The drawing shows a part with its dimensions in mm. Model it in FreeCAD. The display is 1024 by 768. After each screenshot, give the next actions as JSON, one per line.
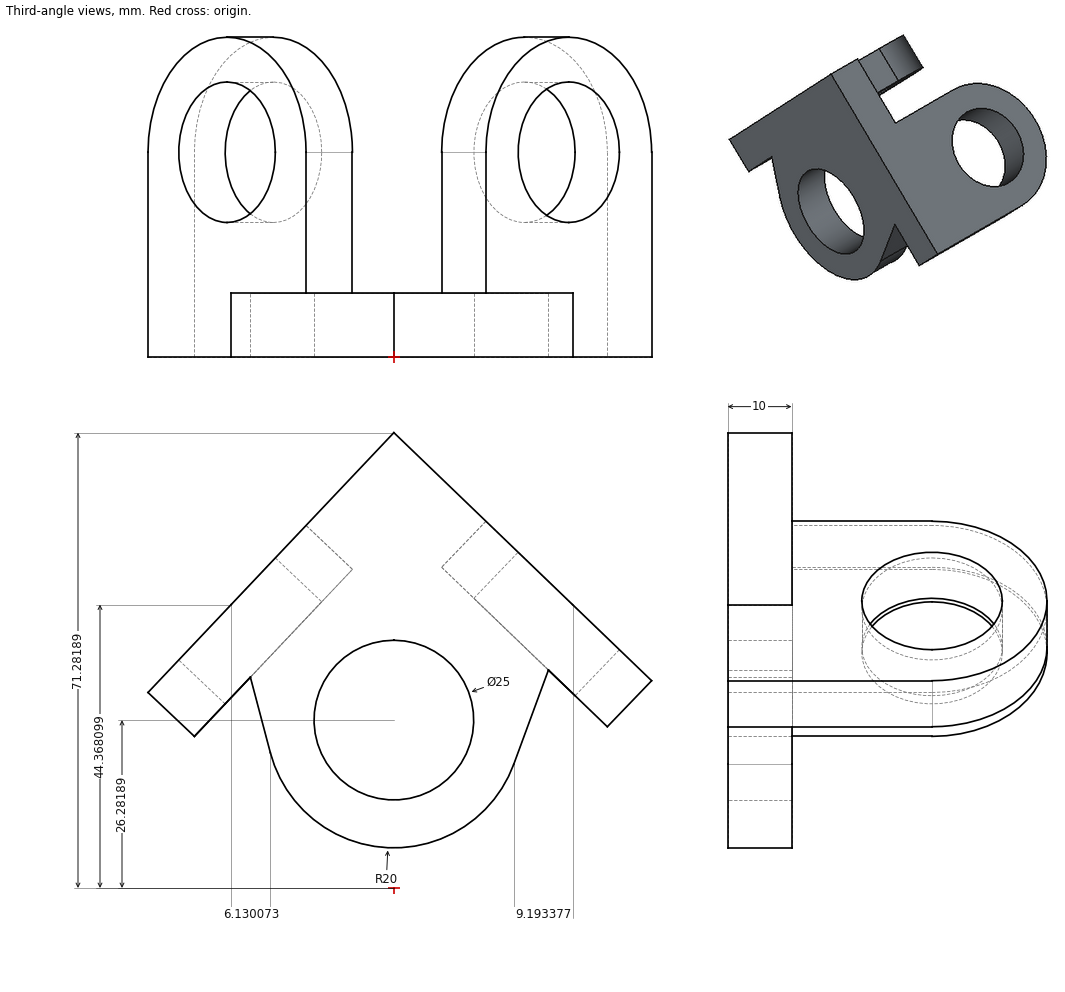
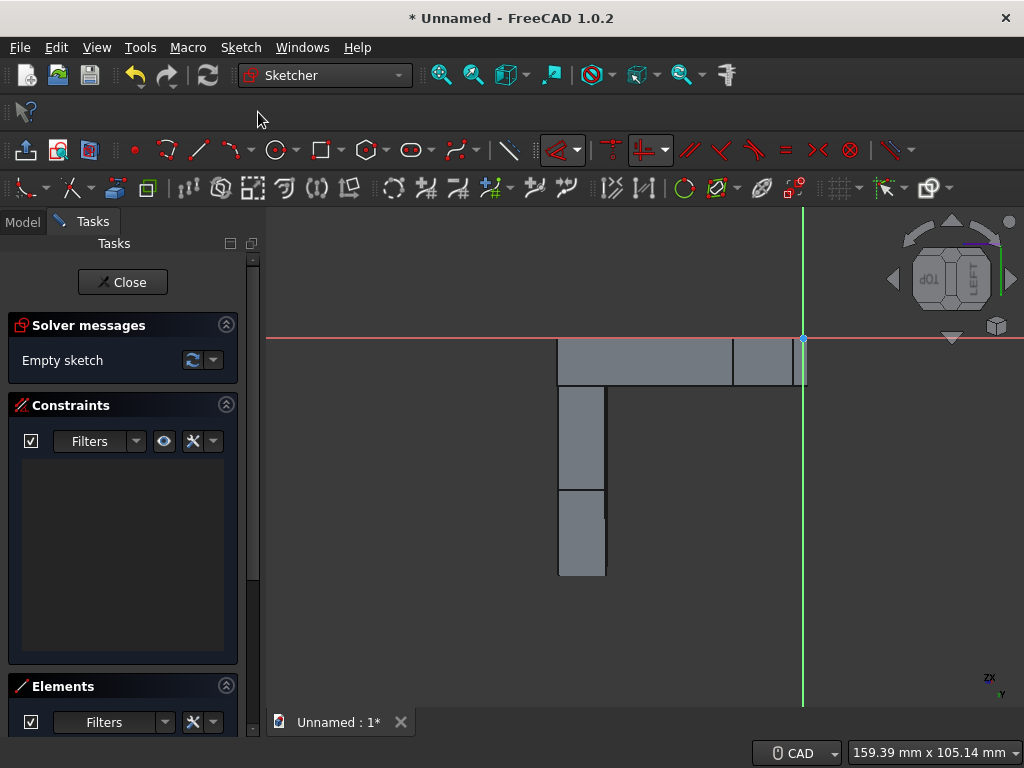
{"action": "left_click", "coordinate": [168, 150]}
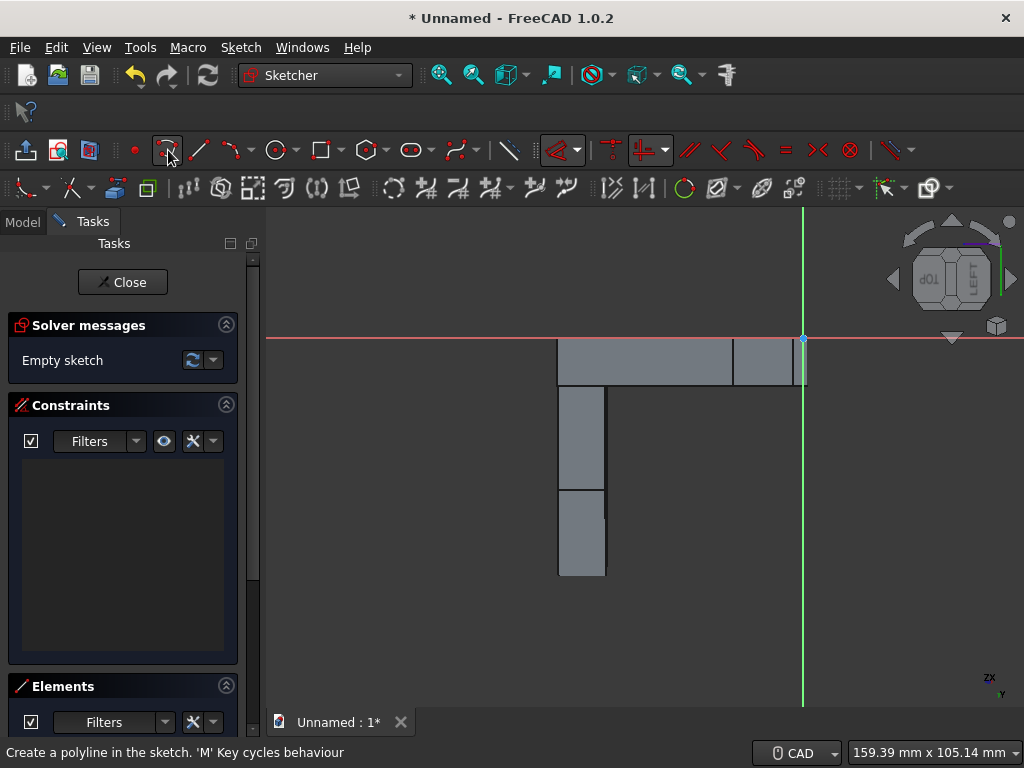
{"action": "left_click", "coordinate": [823, 490]}
{"action": "left_click", "coordinate": [823, 338]}
{"action": "left_click", "coordinate": [652, 347]}
{"action": "left_click", "coordinate": [652, 490]}
{"action": "right_click", "coordinate": [652, 490]}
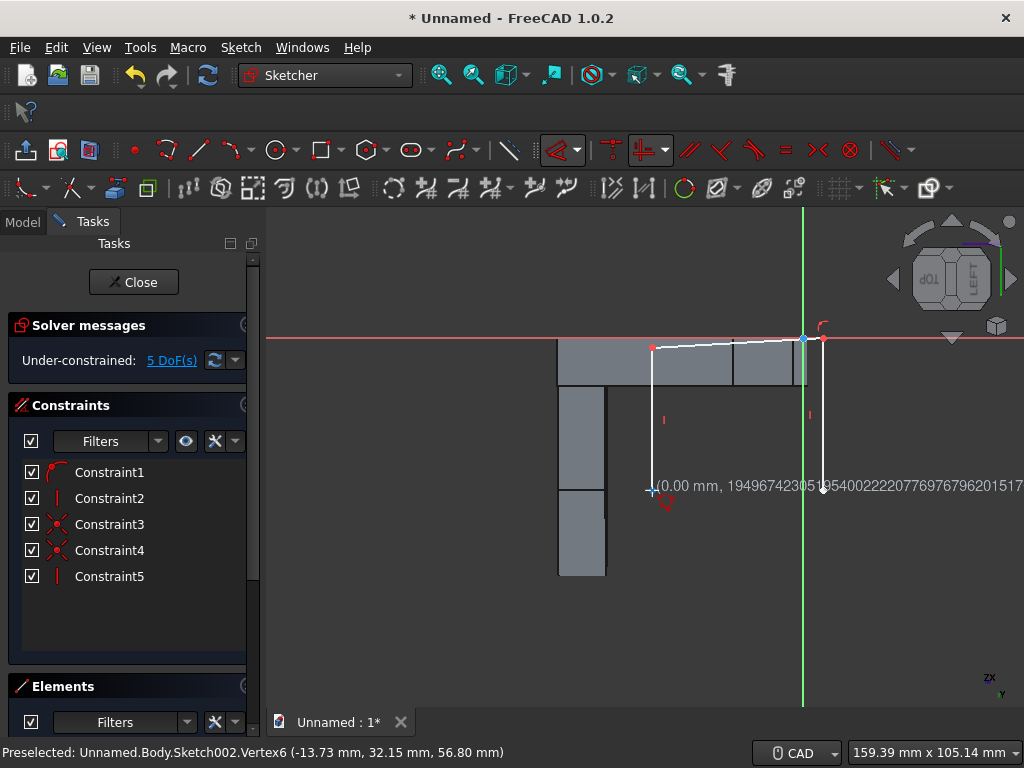
{"action": "left_click", "coordinate": [232, 150]}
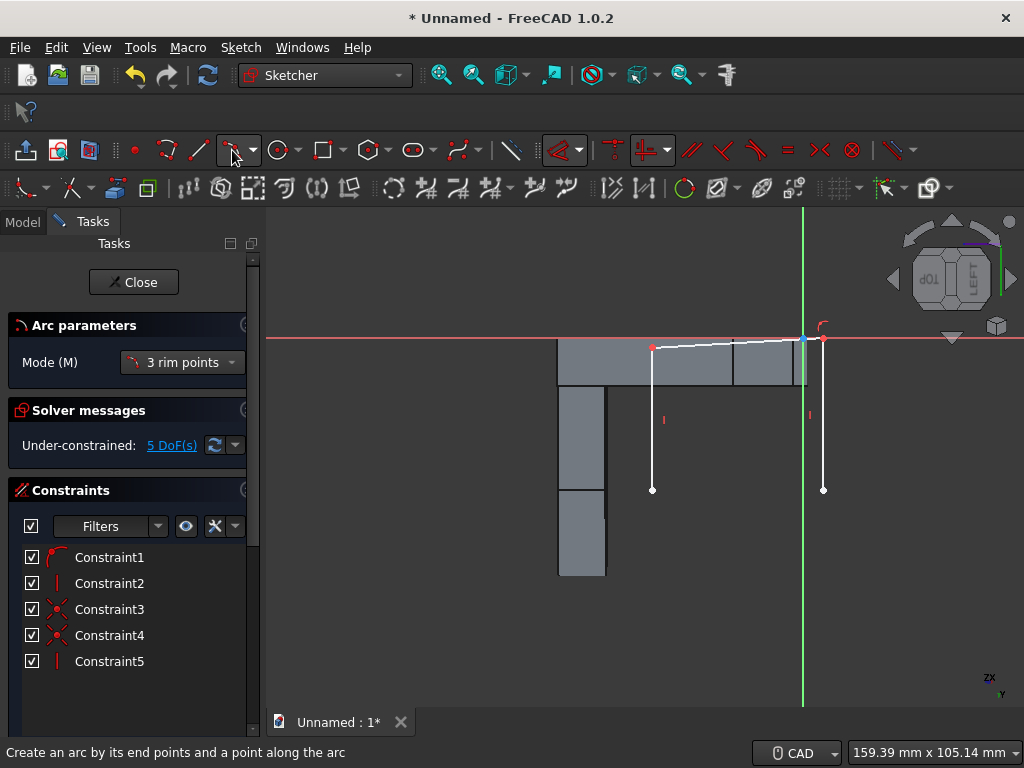
{"action": "left_click", "coordinate": [652, 491]}
{"action": "left_click", "coordinate": [823, 491]}
{"action": "left_click", "coordinate": [738, 576]}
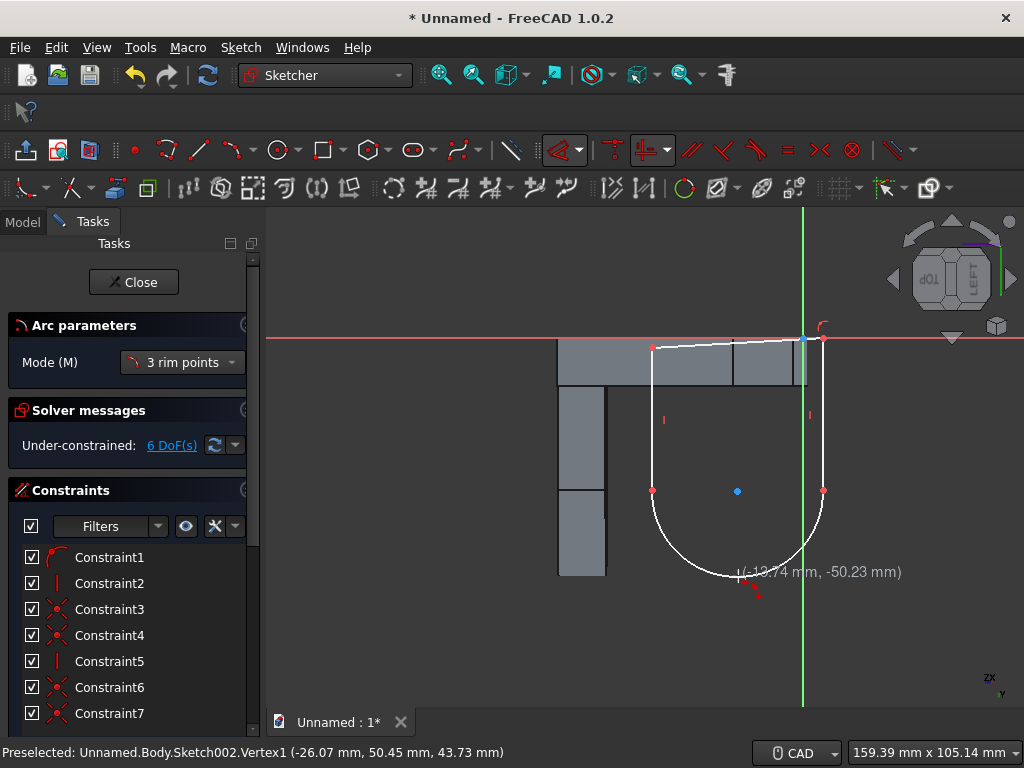
{"action": "left_click", "coordinate": [278, 150]}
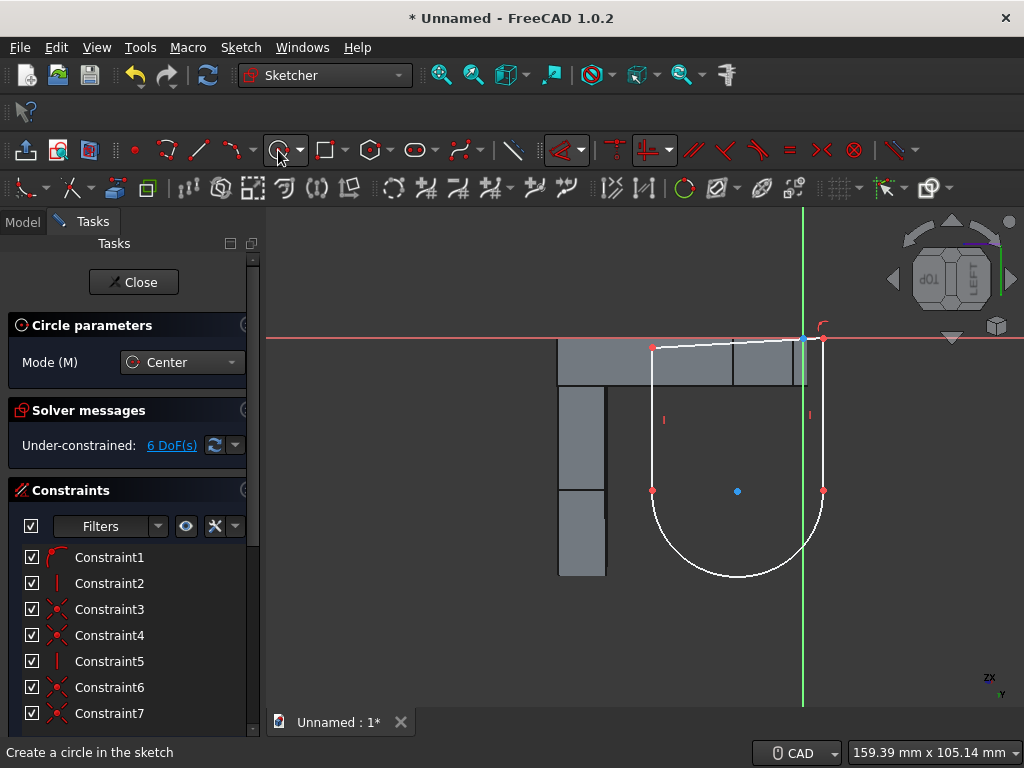
{"action": "left_click", "coordinate": [738, 490]}
{"action": "mouse_move", "coordinate": [775, 453]}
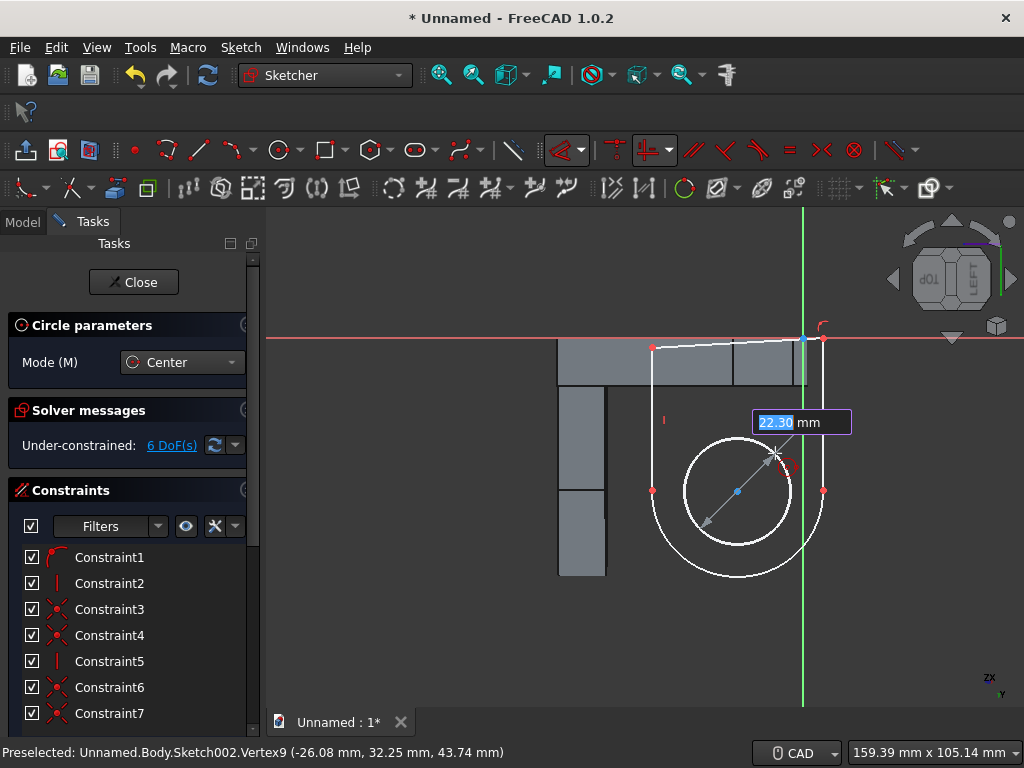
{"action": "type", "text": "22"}
{"action": "key", "text": "Return"}
{"action": "key", "text": "Escape"}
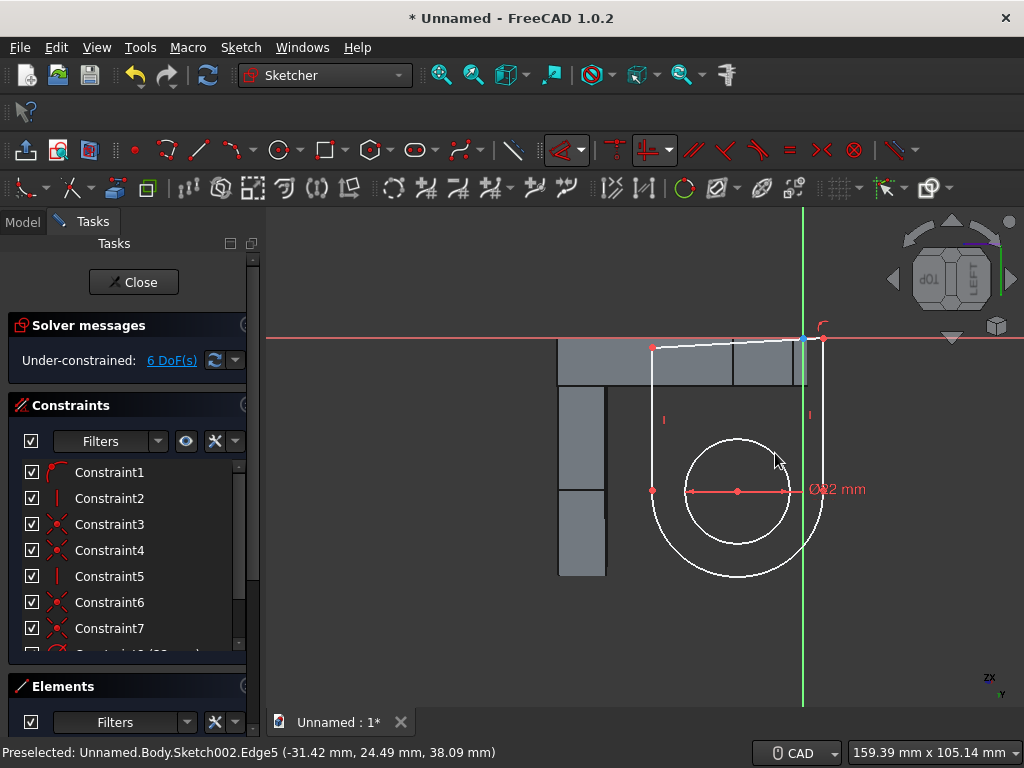
{"action": "left_click", "coordinate": [823, 445]}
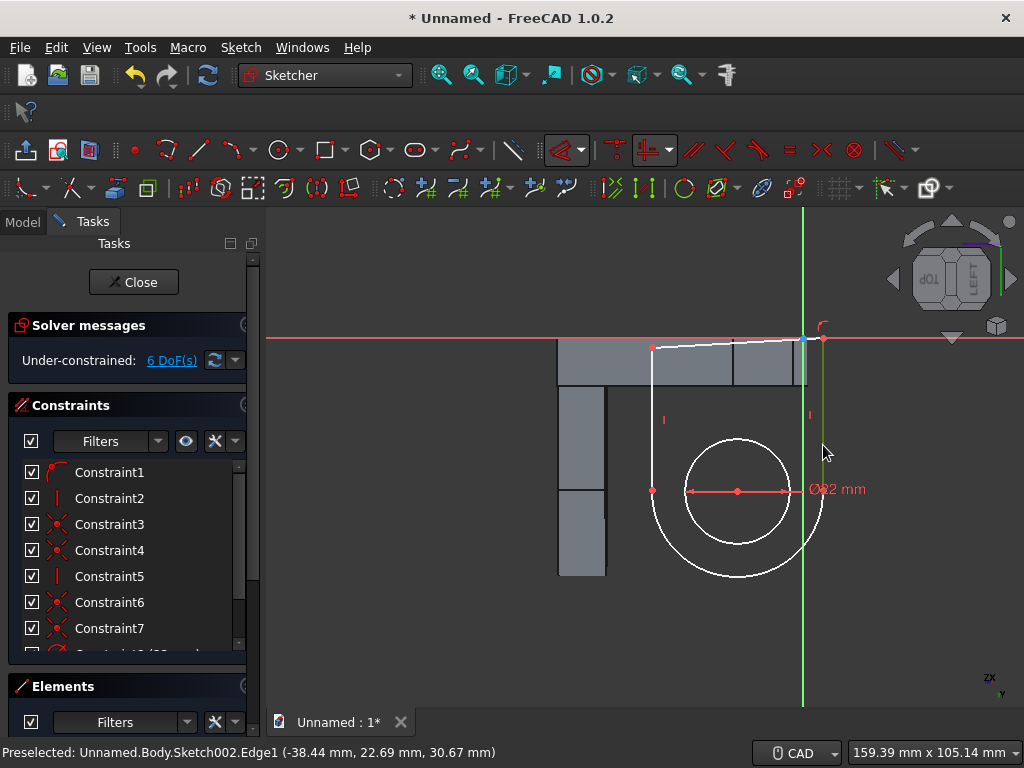
{"action": "left_click", "coordinate": [687, 561]}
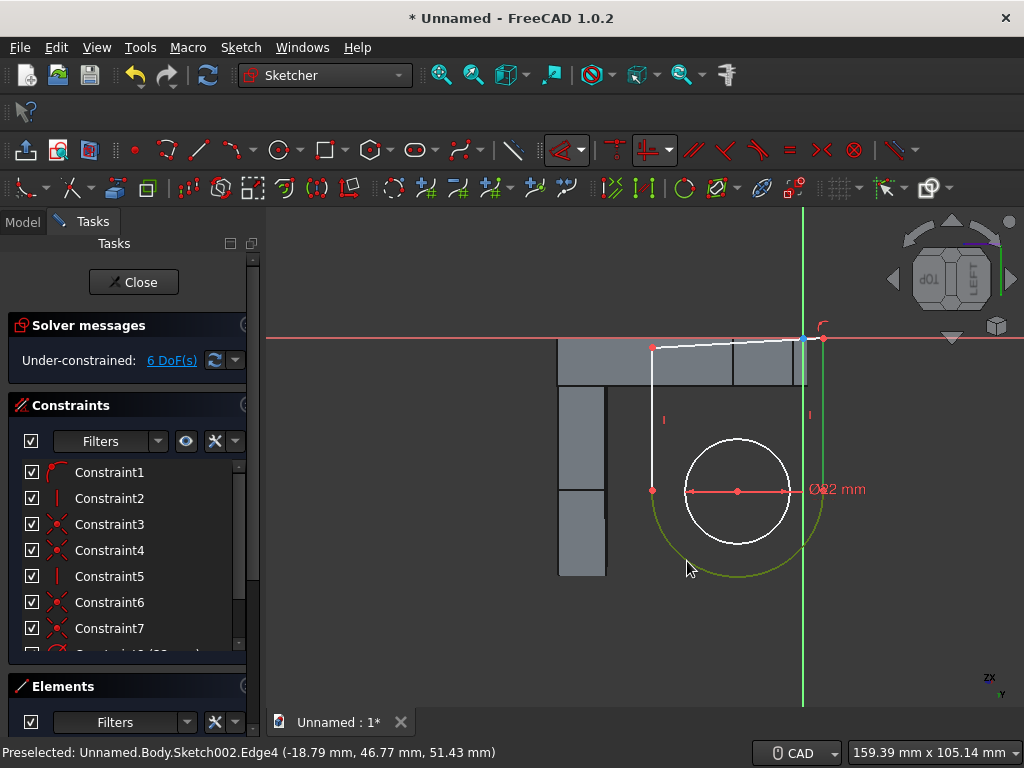
{"action": "left_click", "coordinate": [758, 150]}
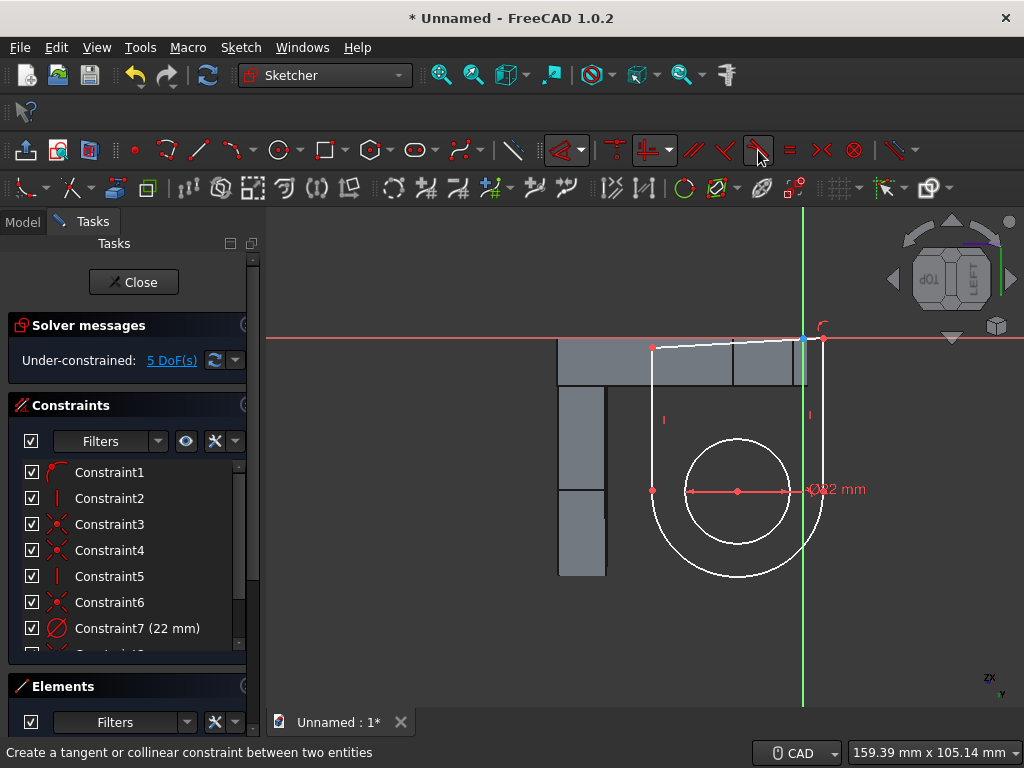
{"action": "left_click", "coordinate": [652, 391]}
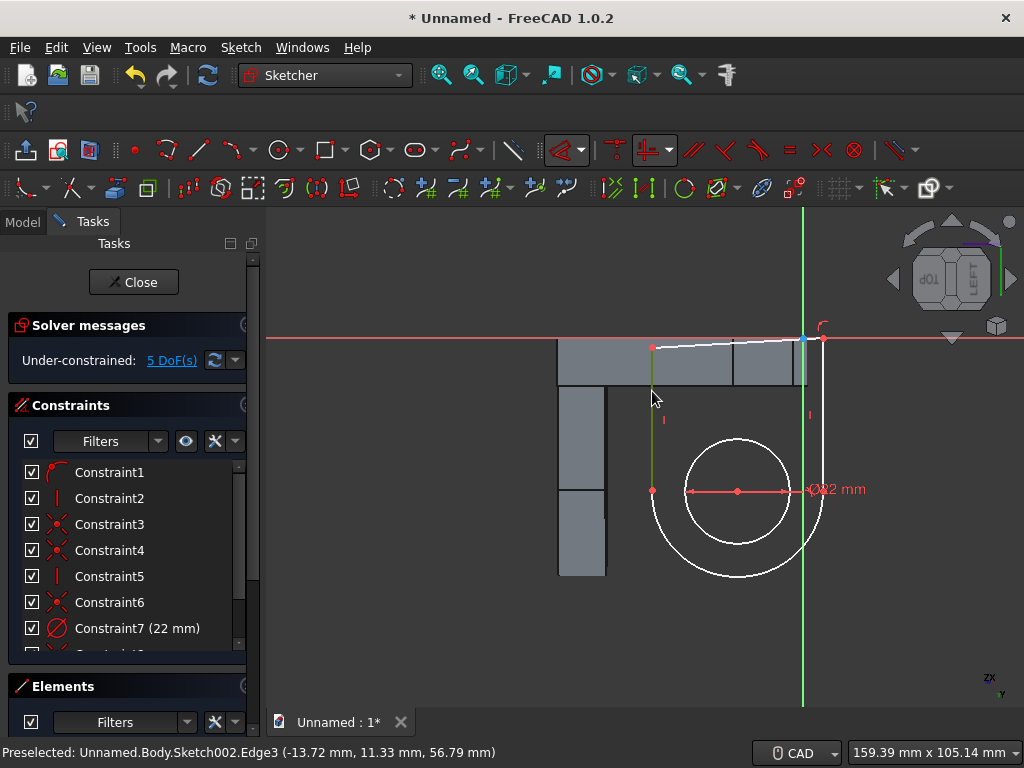
{"action": "left_click", "coordinate": [687, 560]}